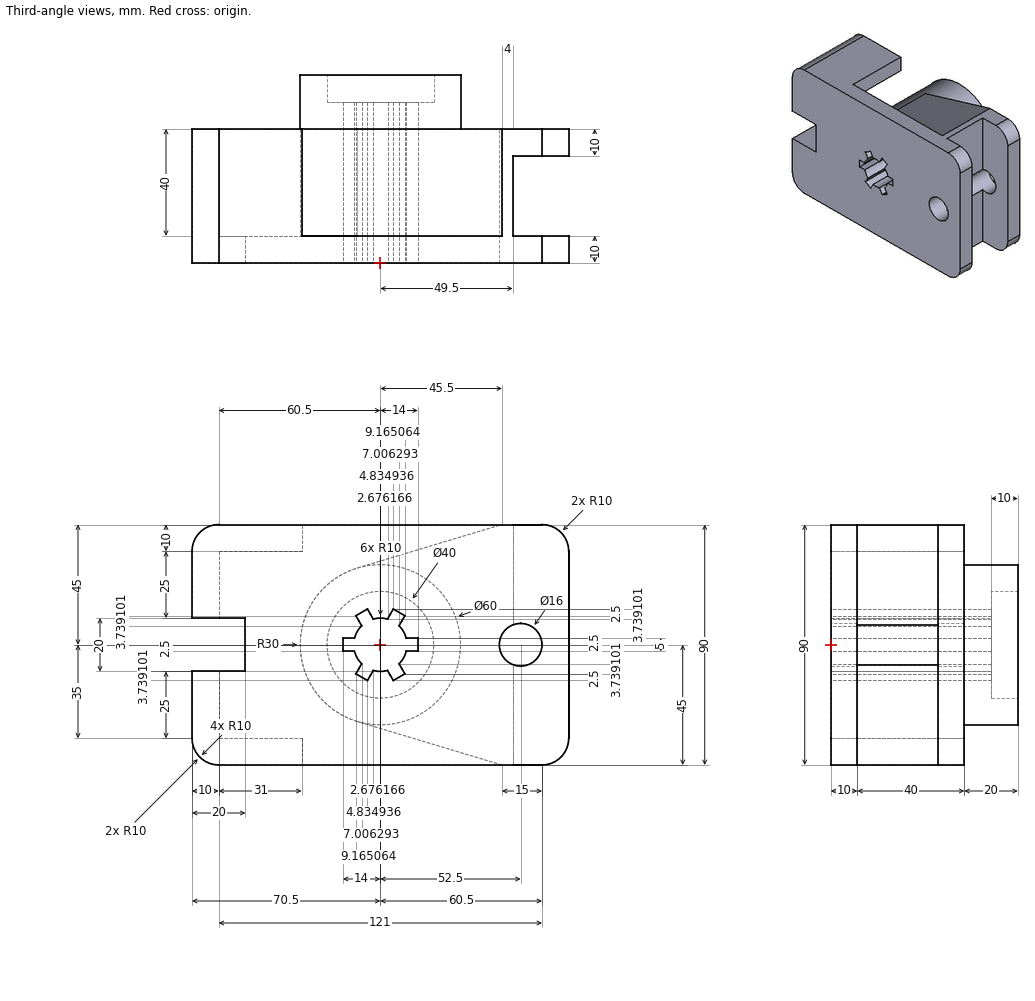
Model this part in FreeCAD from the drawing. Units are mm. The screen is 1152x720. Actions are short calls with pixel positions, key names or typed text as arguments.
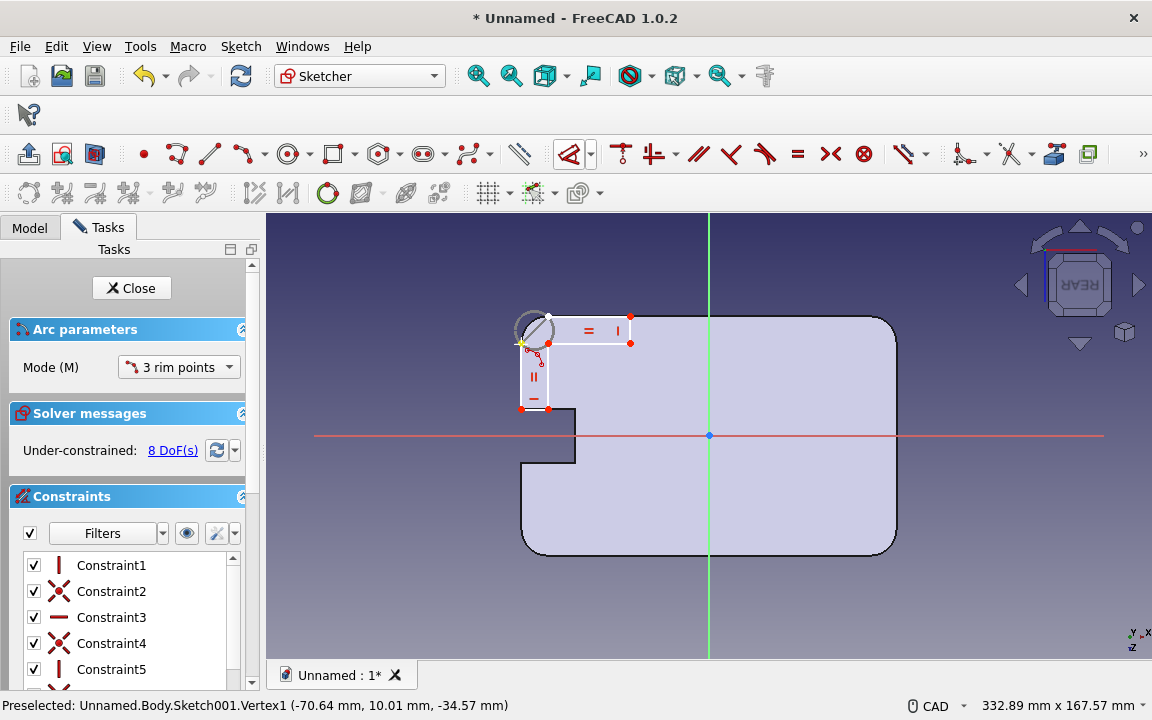
scroll(529, 324, up, 4)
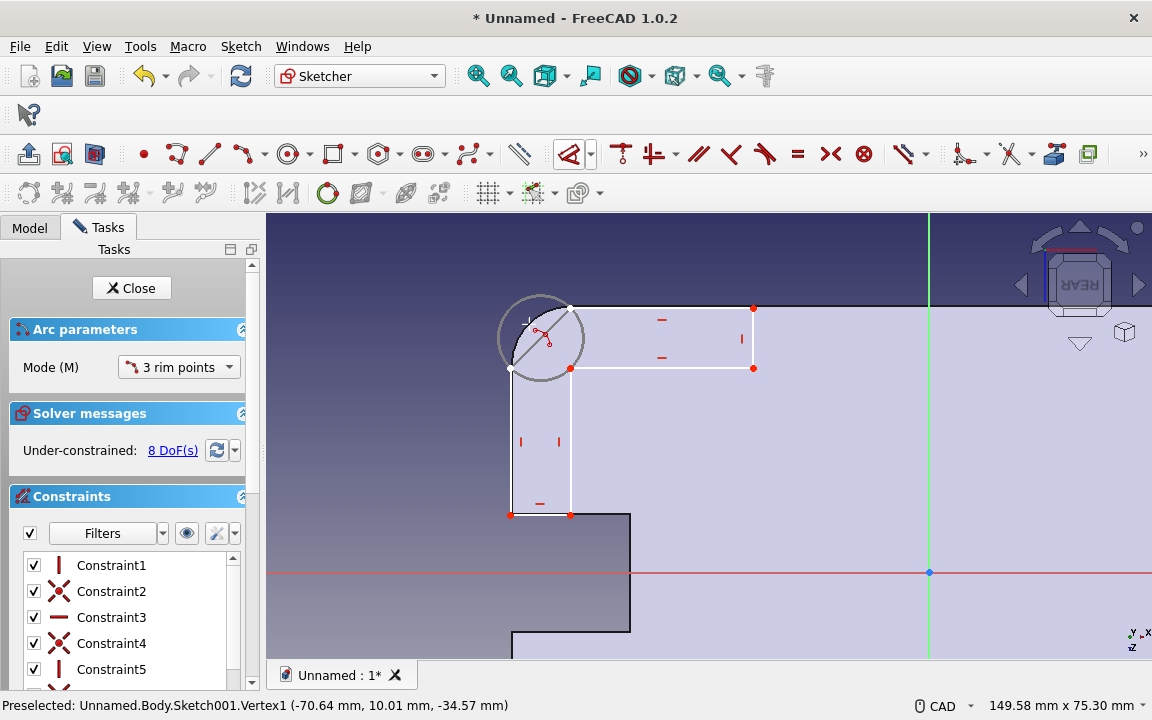
click(529, 324)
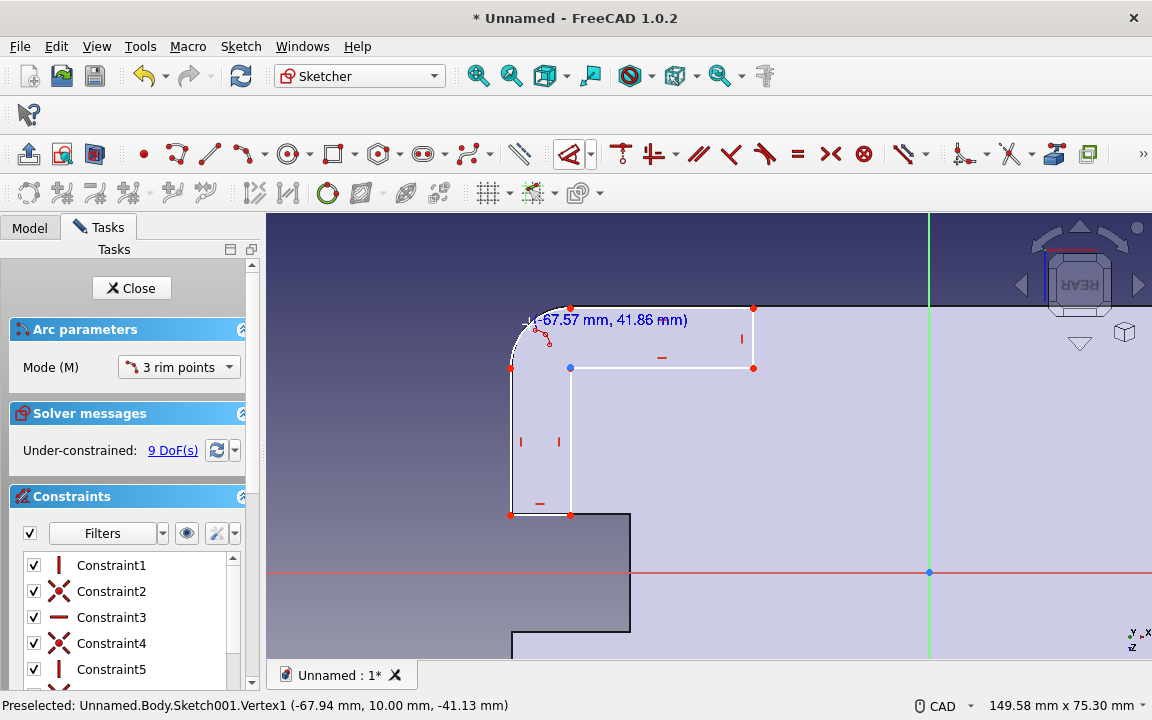
click(177, 154)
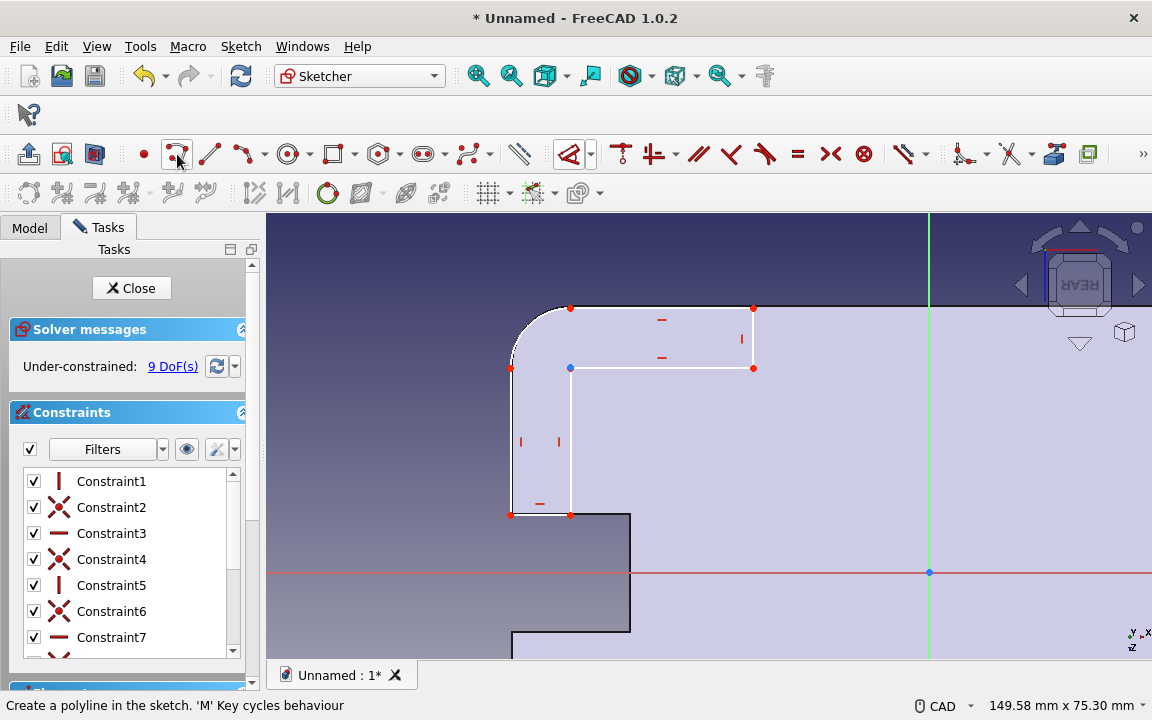
scroll(543, 269, down, 3)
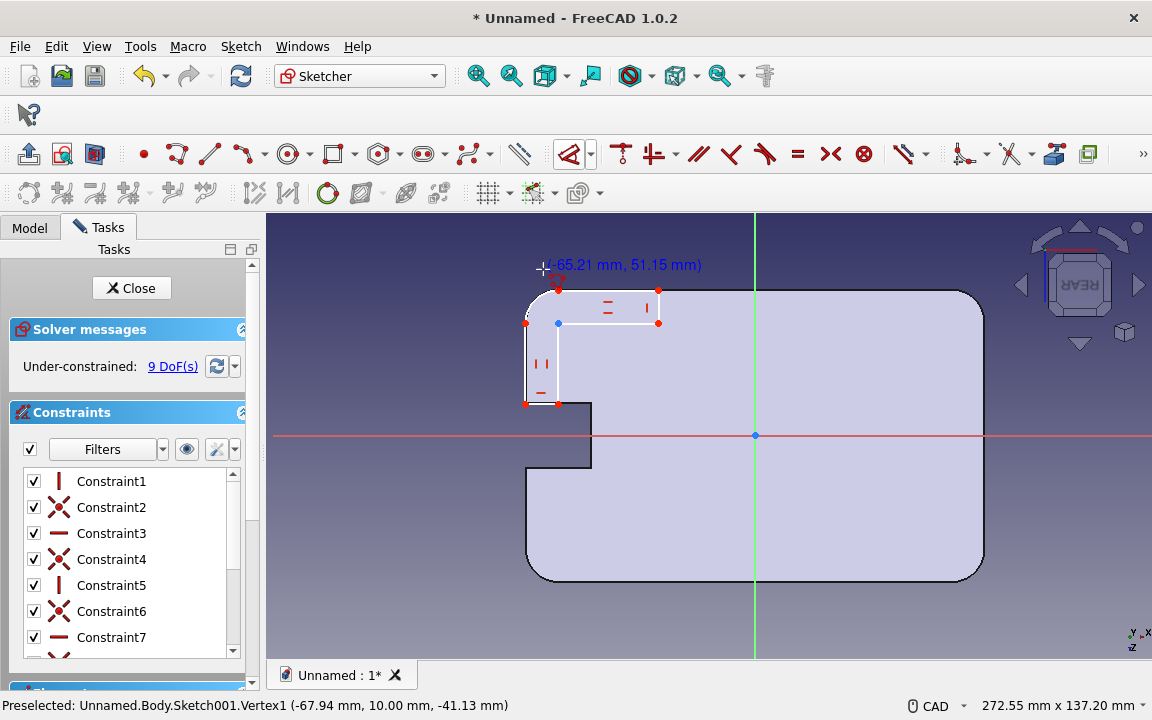
click(558, 582)
click(659, 582)
click(659, 550)
click(558, 550)
click(558, 468)
click(526, 468)
click(526, 550)
right_click(526, 550)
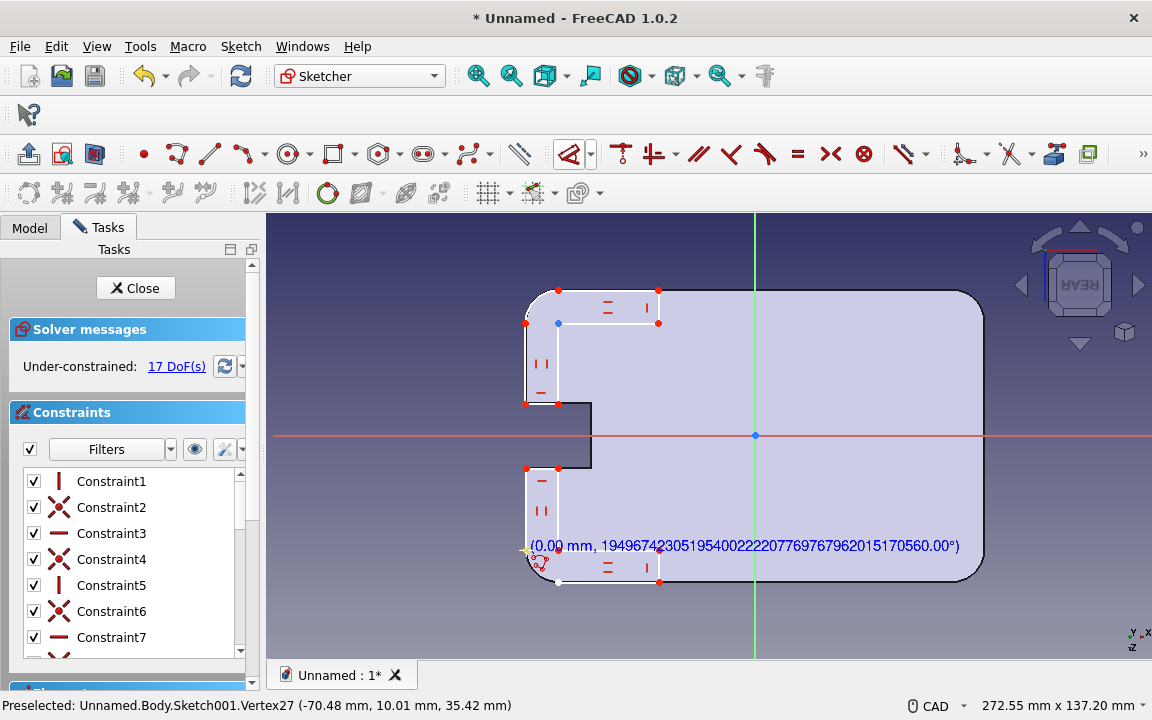
click(242, 154)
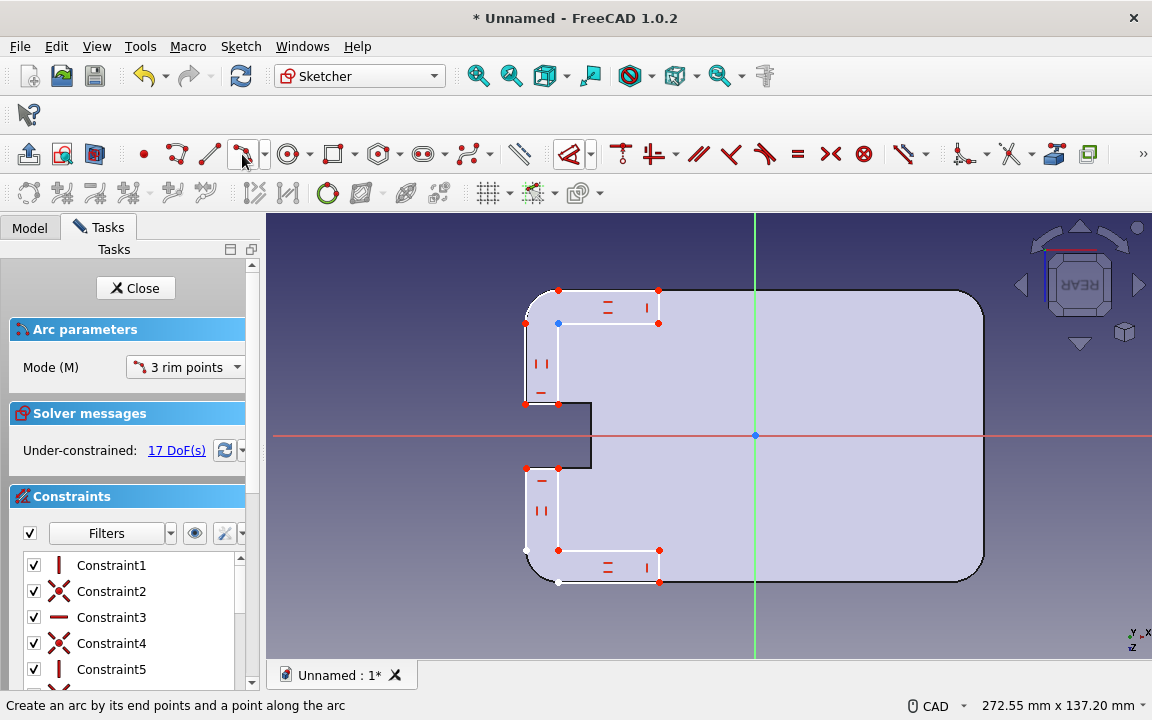
click(526, 551)
click(558, 583)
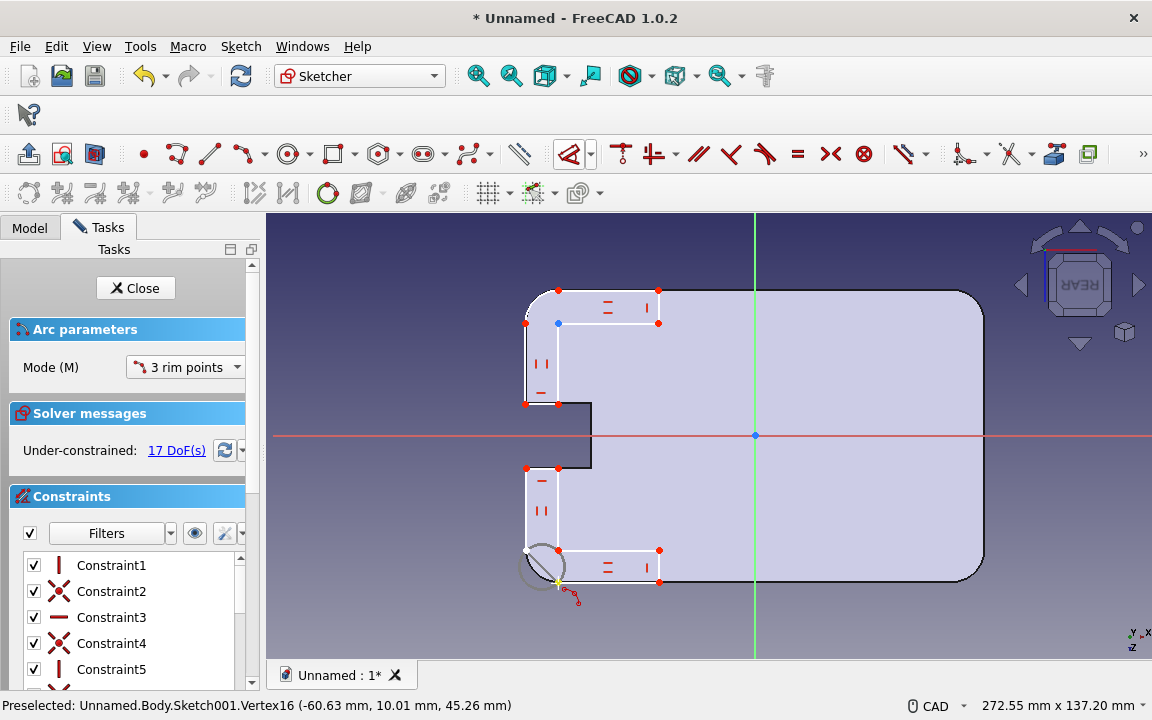
scroll(535, 573, up, 3)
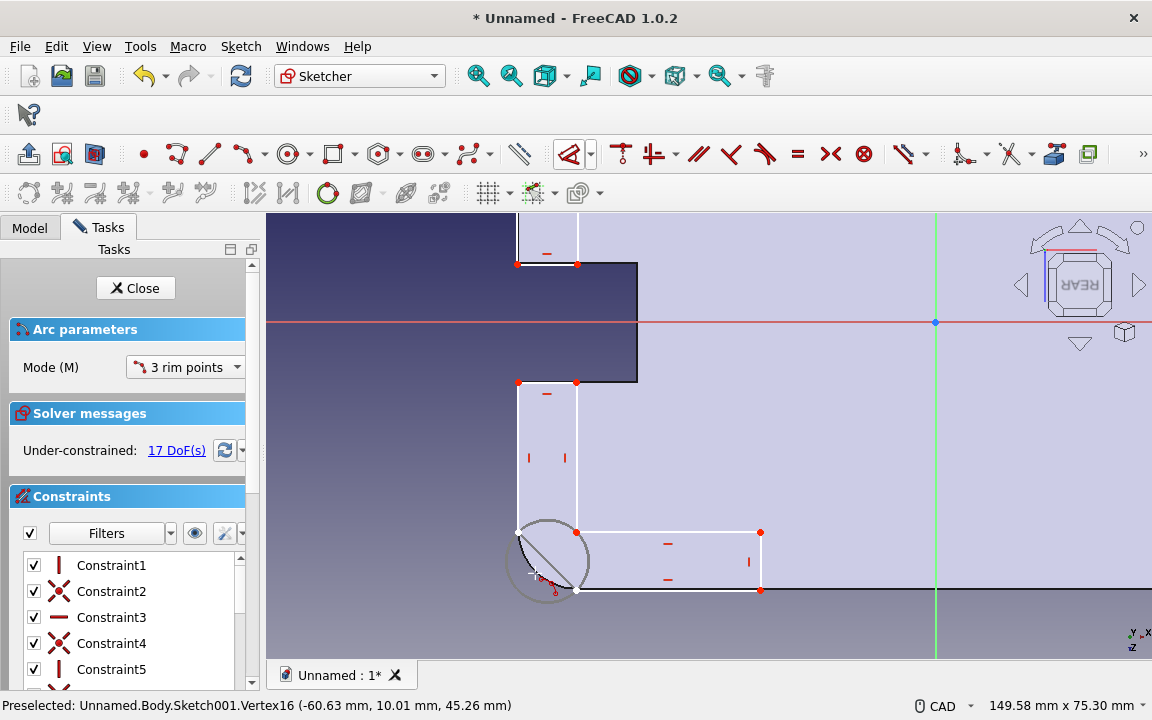
click(536, 572)
key(Escape)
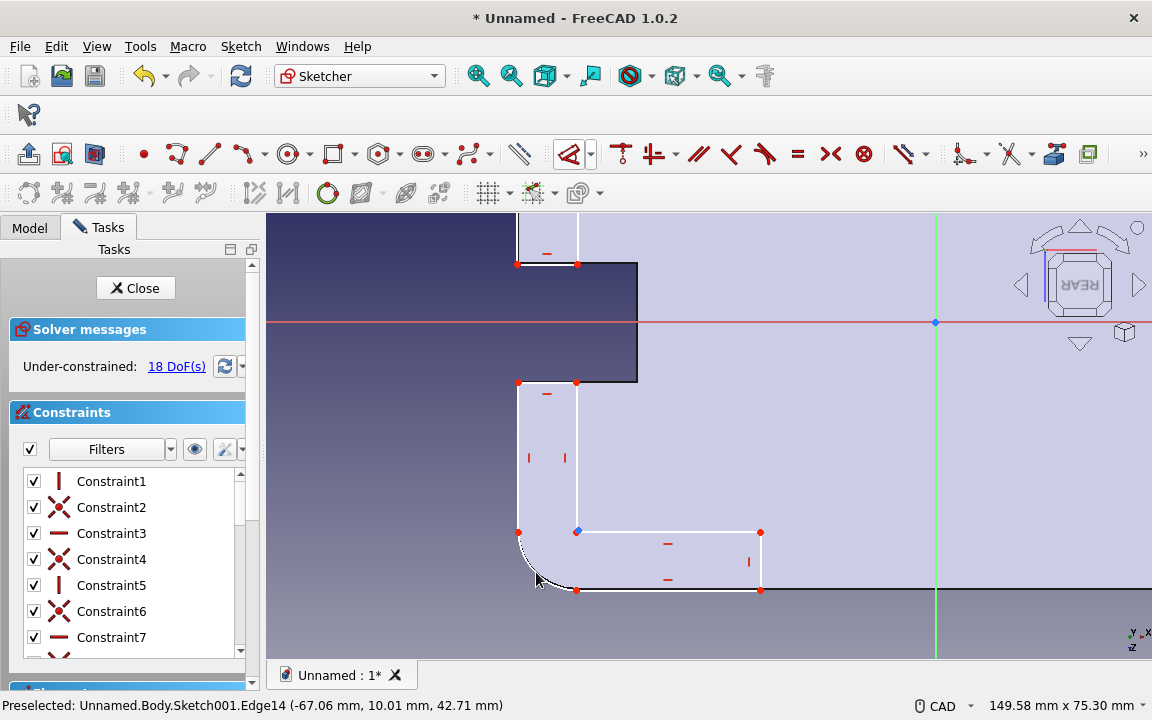
scroll(535, 574, down, 3)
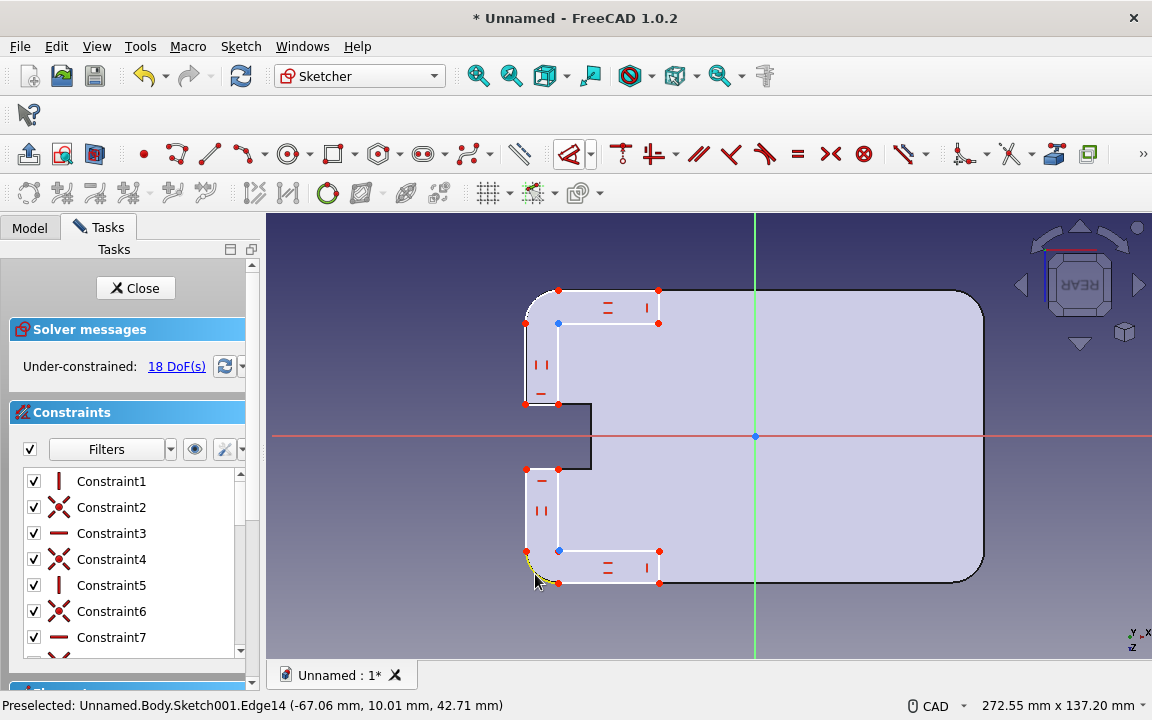
click(525, 348)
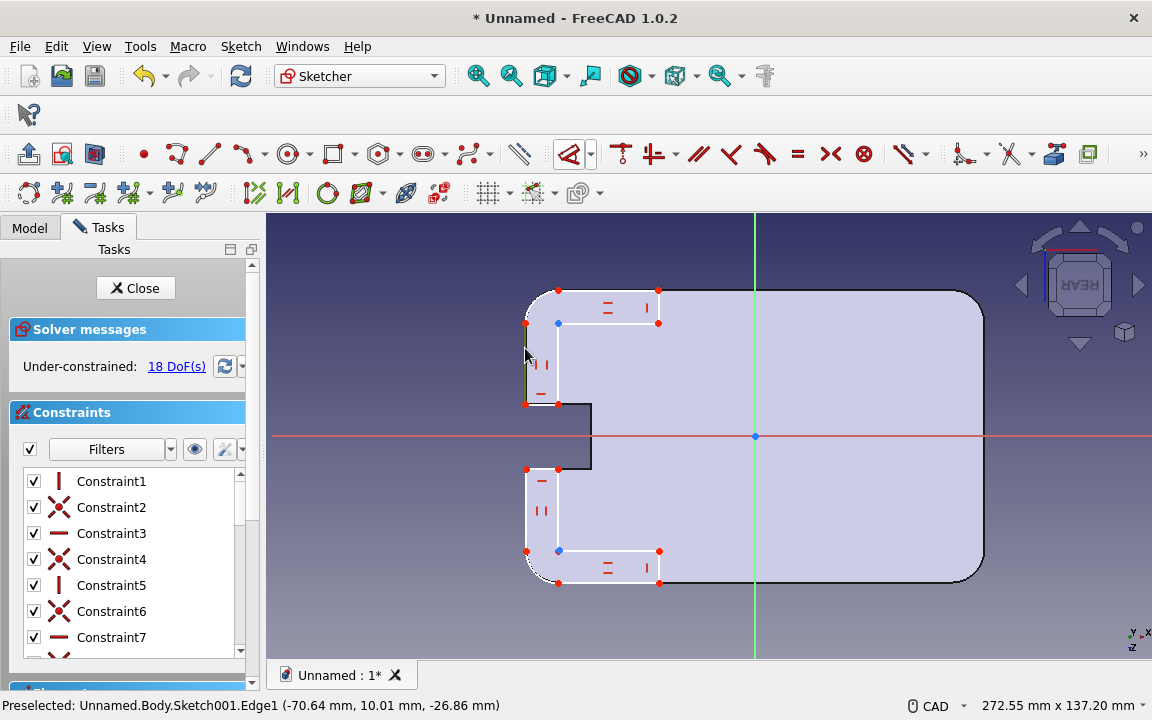
click(543, 295)